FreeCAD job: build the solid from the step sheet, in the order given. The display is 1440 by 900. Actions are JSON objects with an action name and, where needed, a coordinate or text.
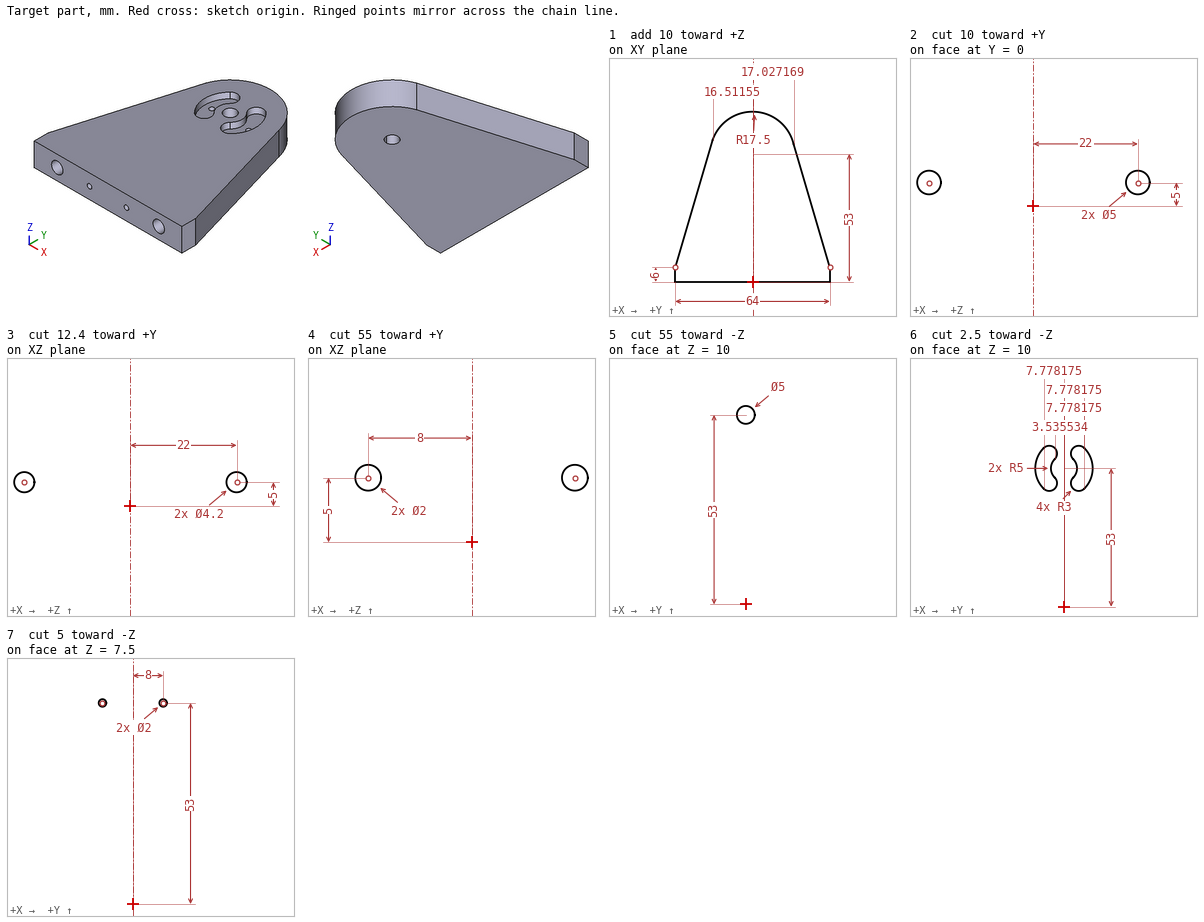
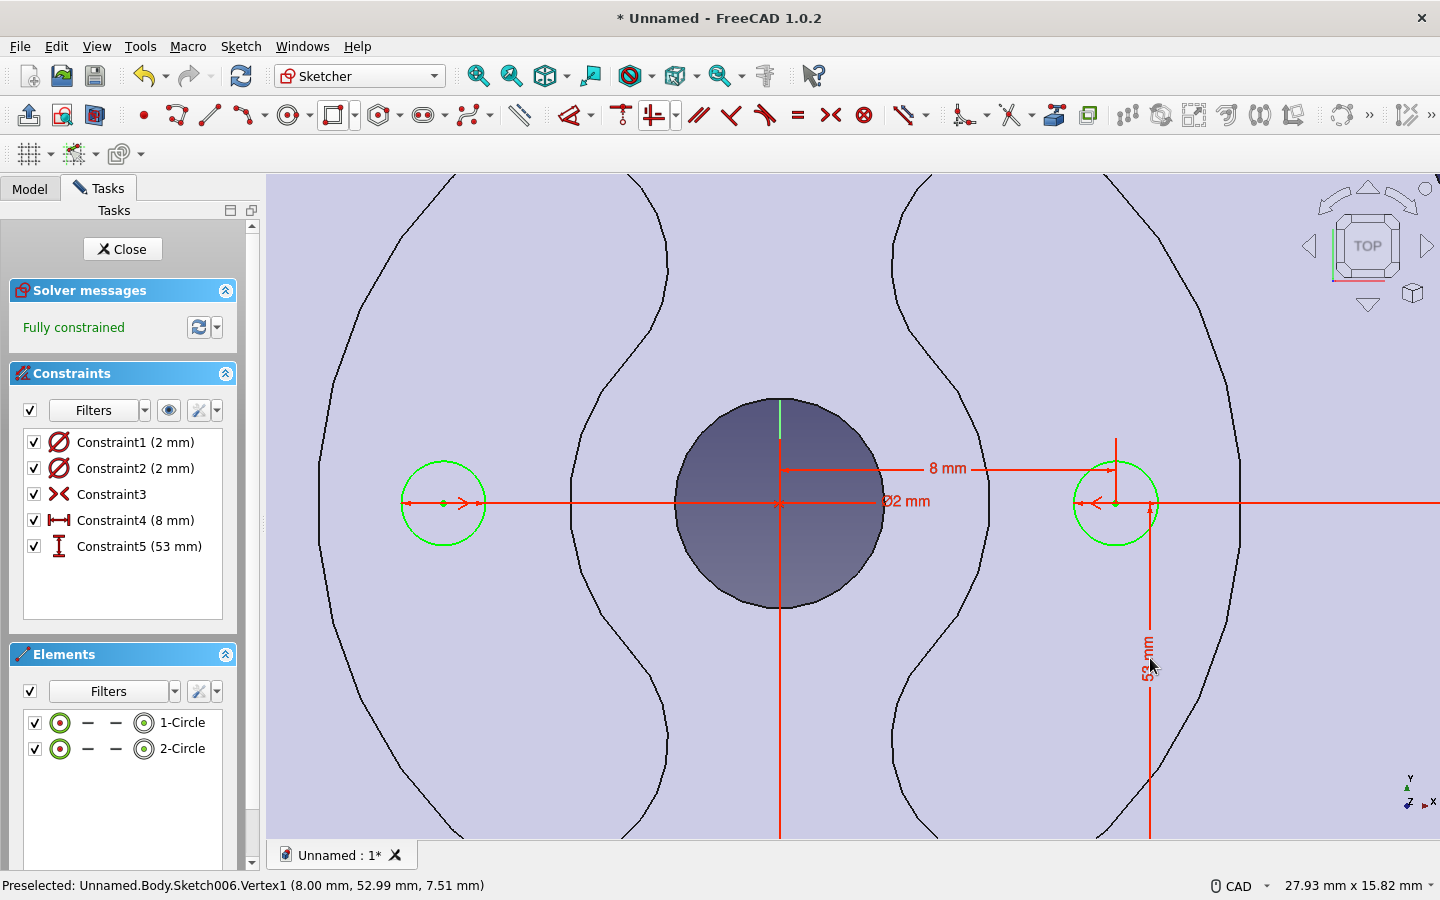
{"action": "left_click", "coordinate": [123, 249]}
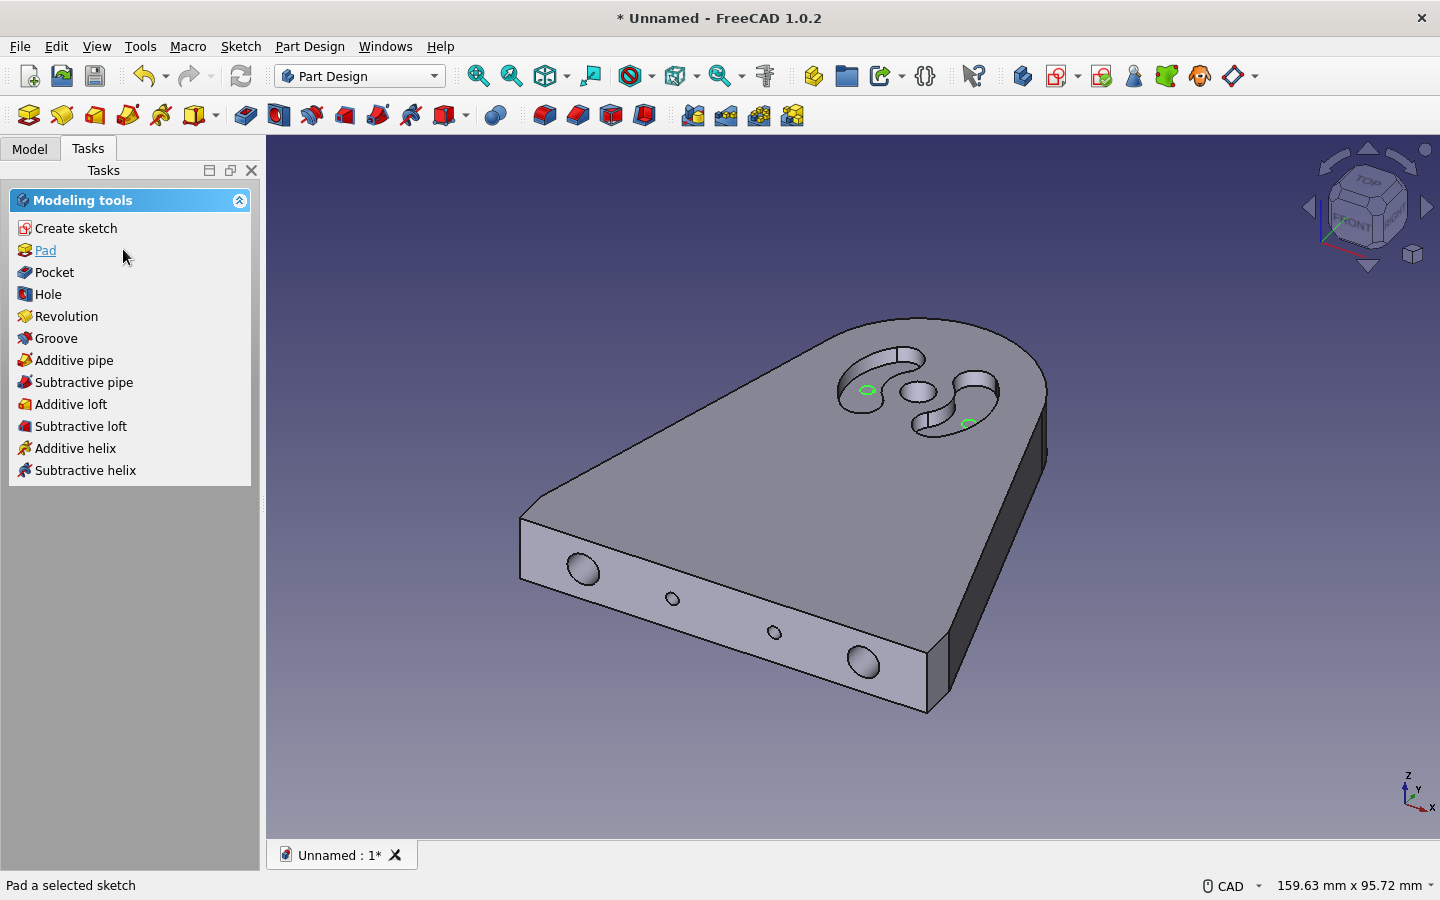
{"action": "left_click", "coordinate": [246, 116]}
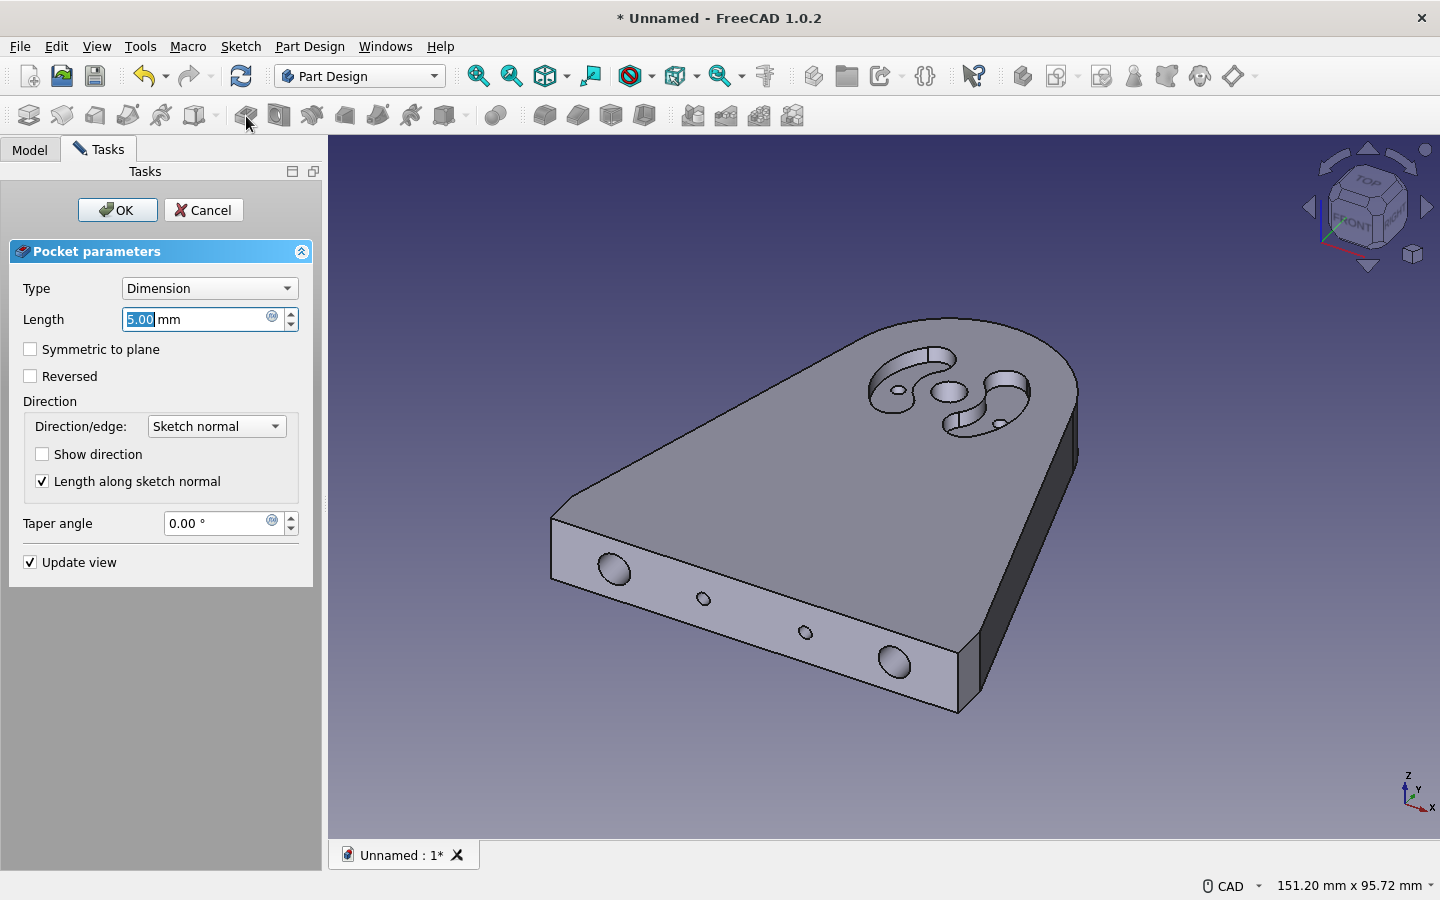
{"action": "type", "text": "5"}
{"action": "key", "text": "Tab"}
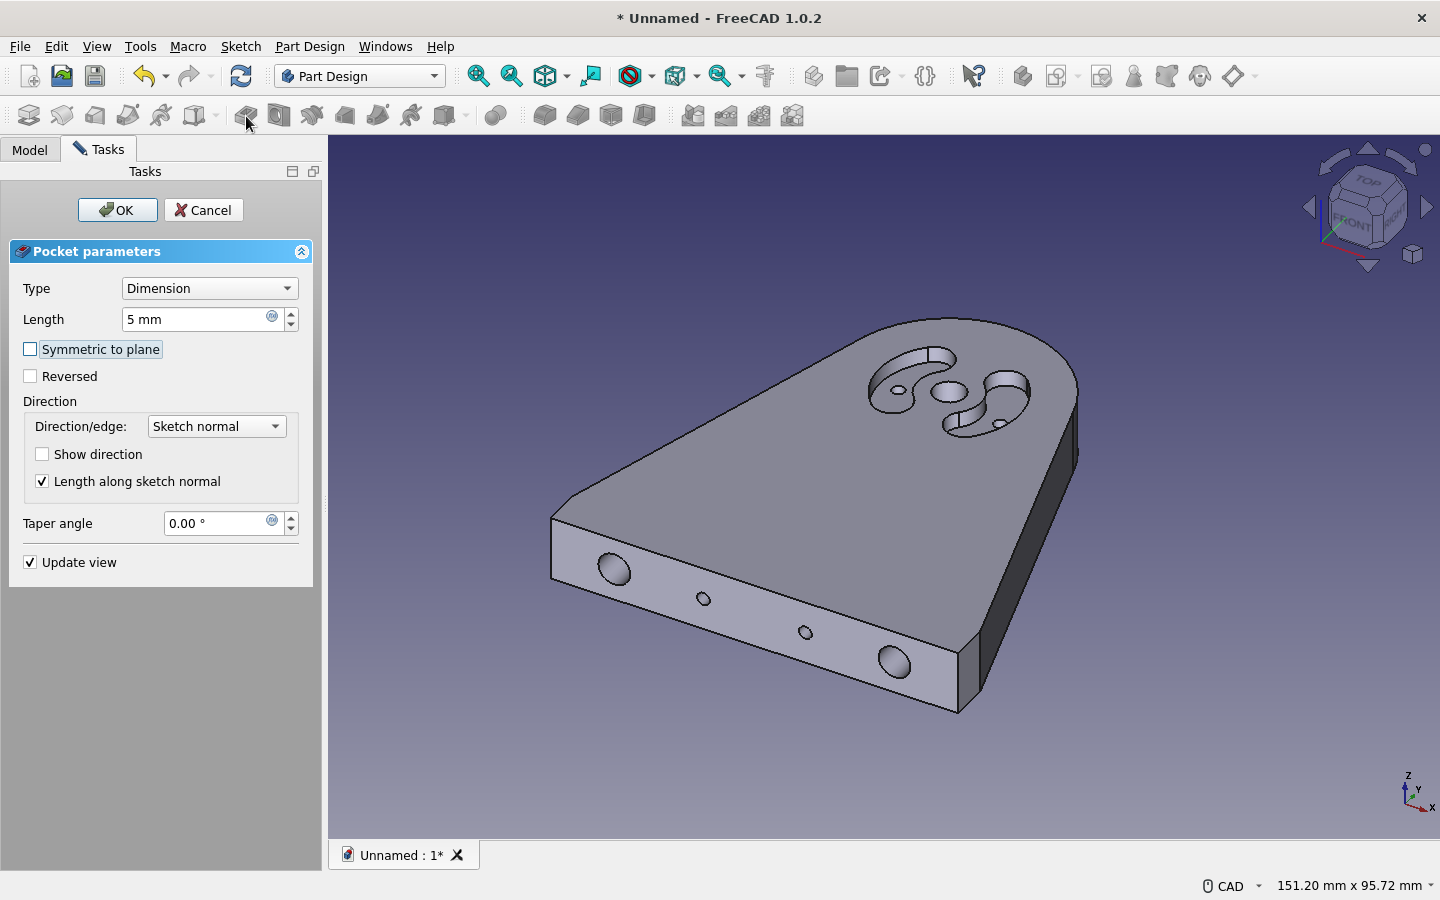
{"action": "left_click", "coordinate": [118, 210]}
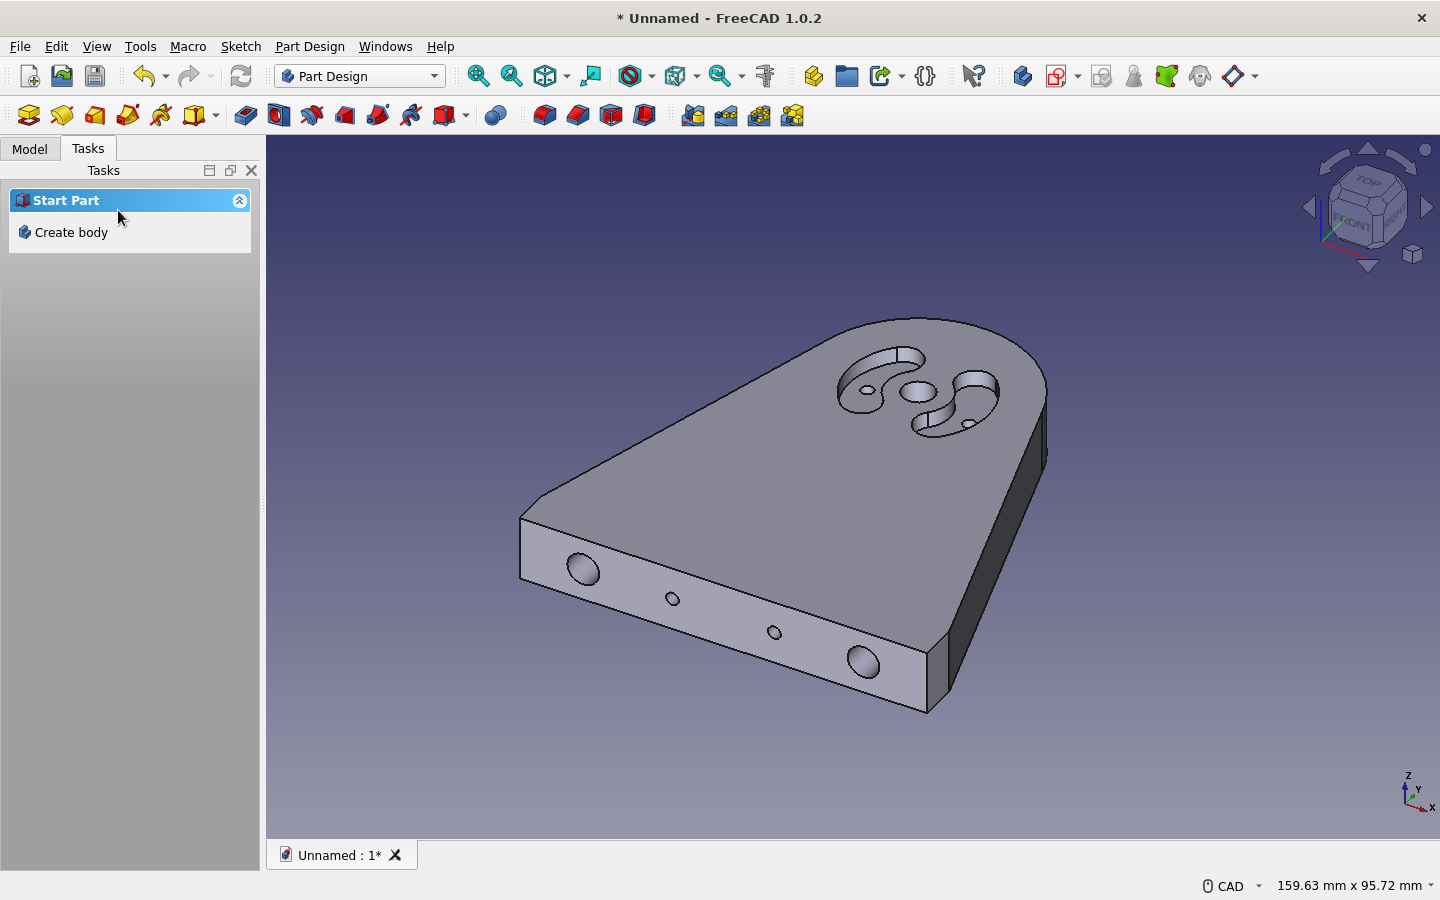
{"action": "key", "text": "0"}